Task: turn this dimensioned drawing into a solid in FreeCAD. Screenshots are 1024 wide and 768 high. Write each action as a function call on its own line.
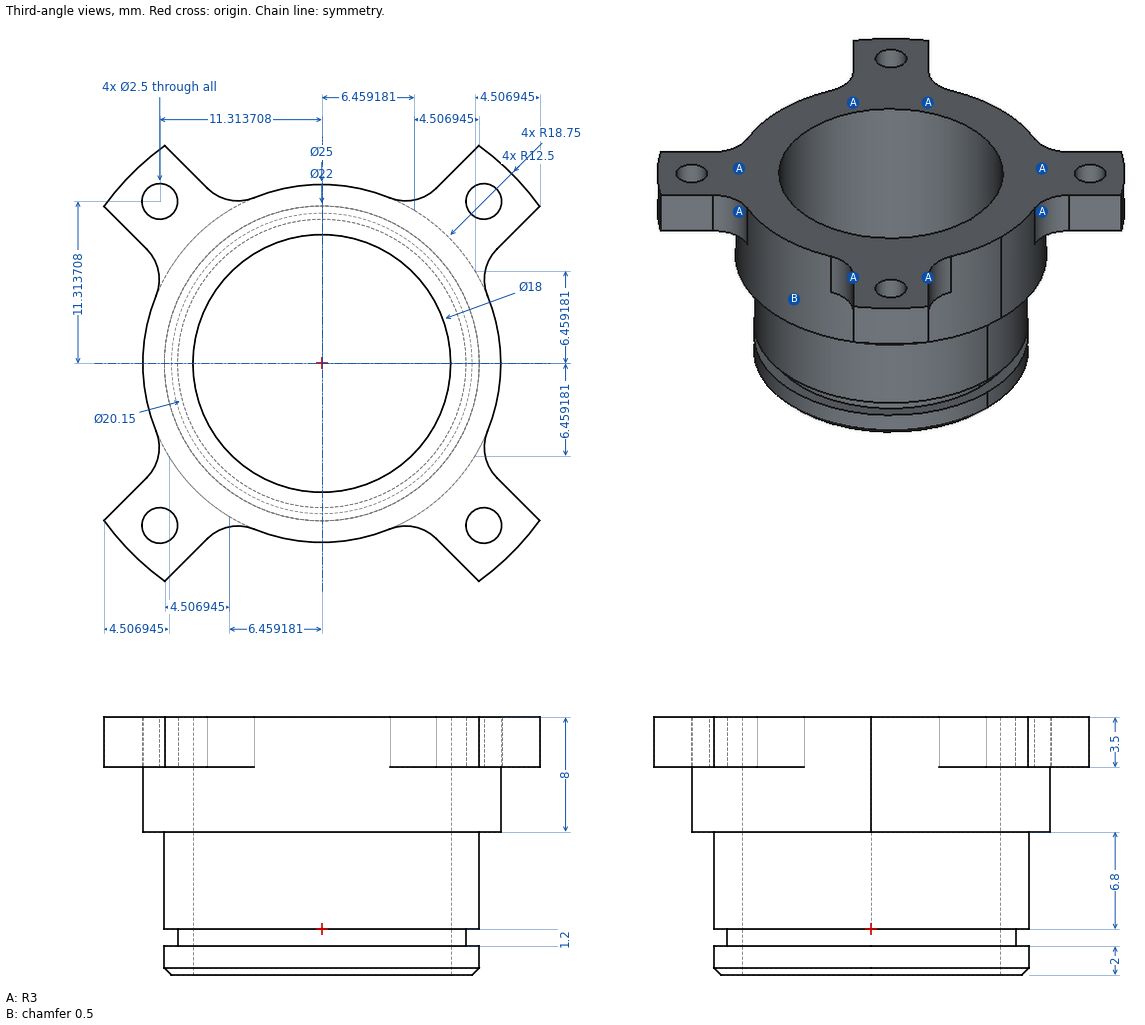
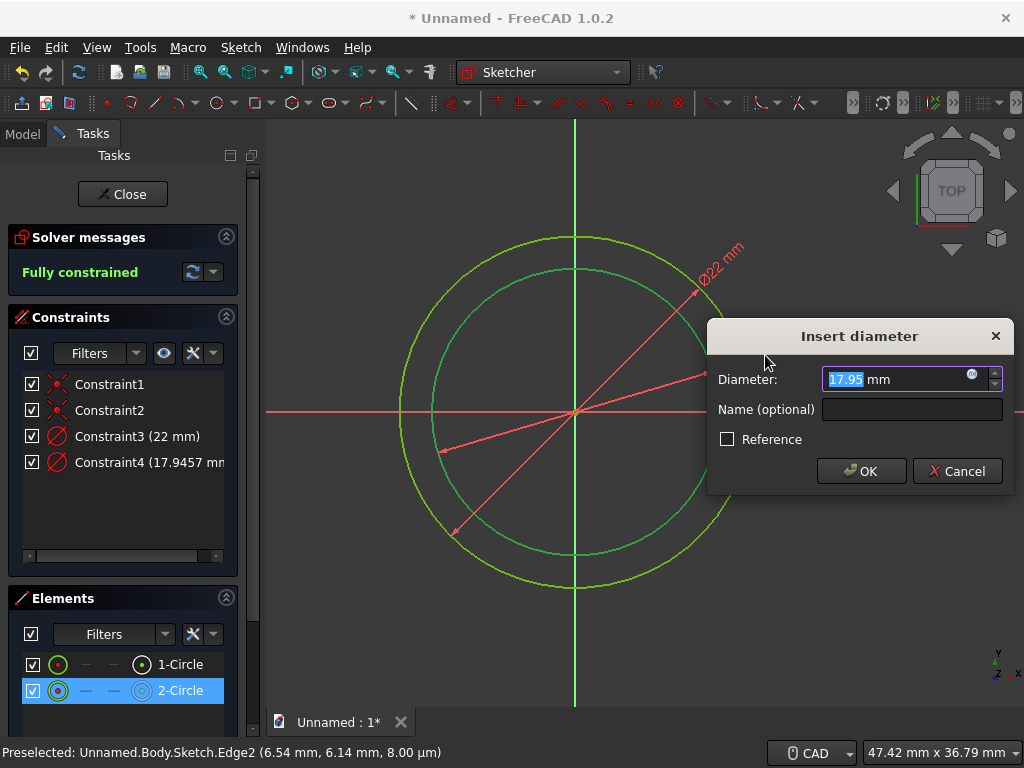
text(18)
key(Return)
key(Escape)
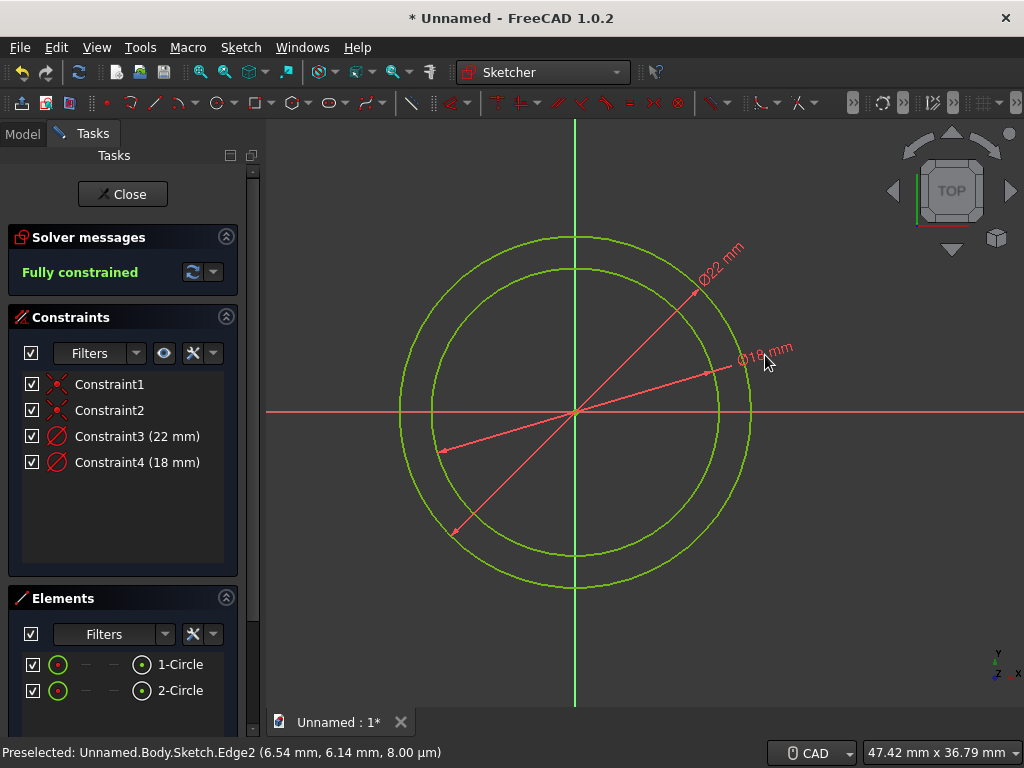
click(123, 194)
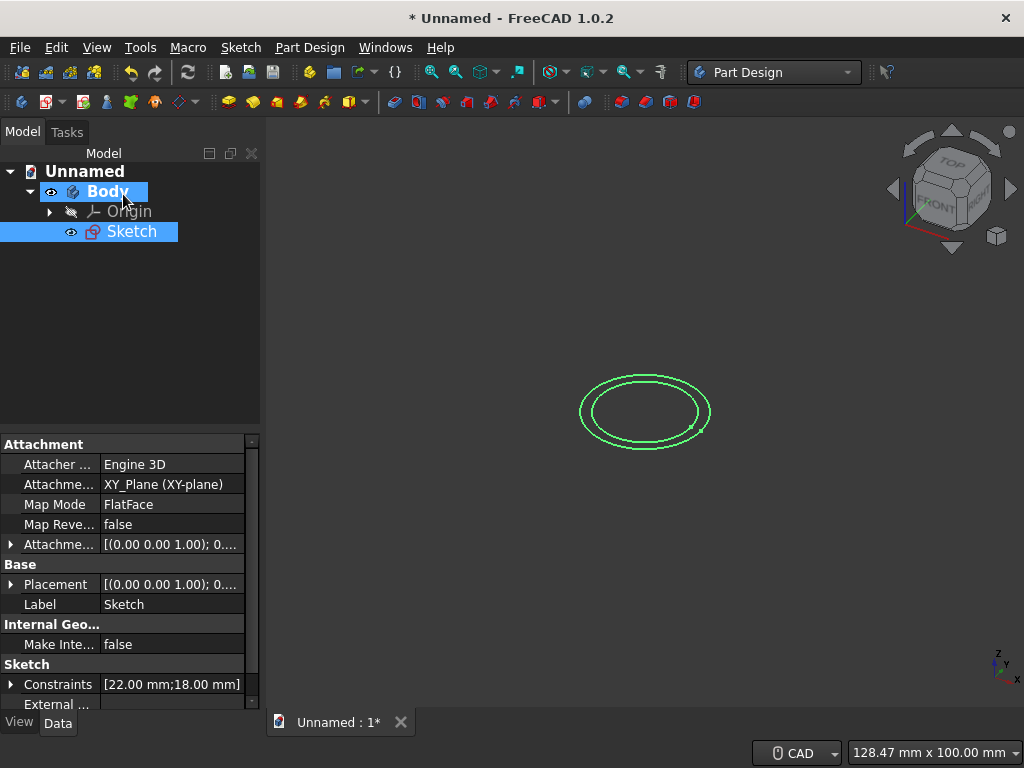
click(230, 102)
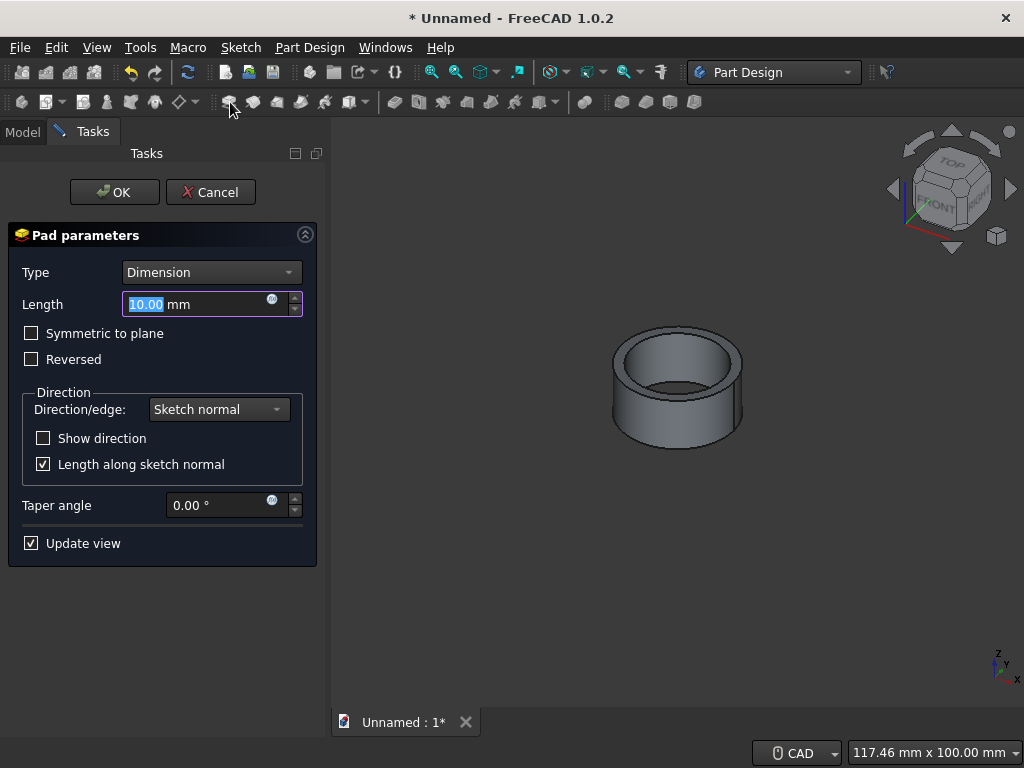
text(6.8)
key(Tab)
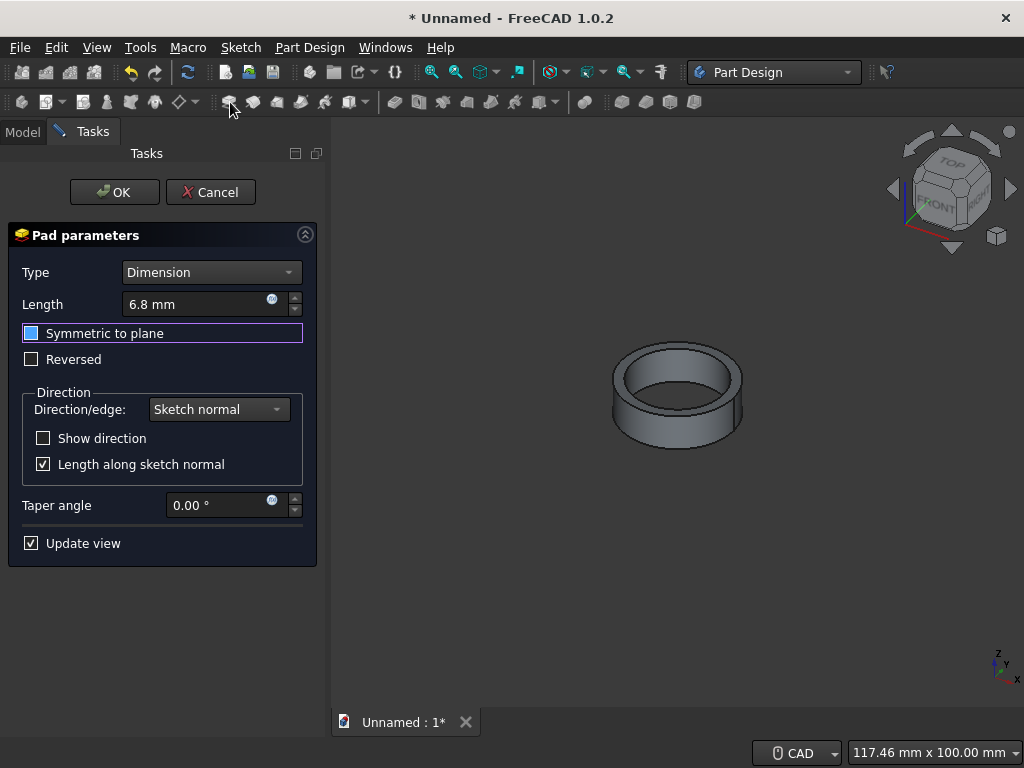
click(115, 192)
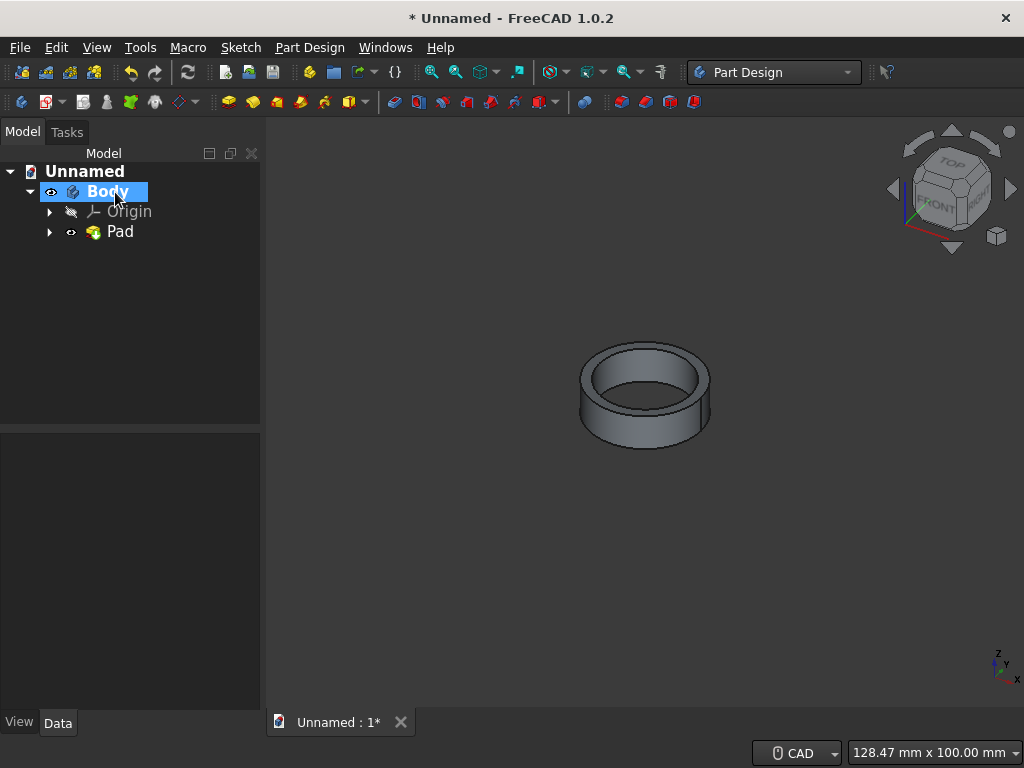
click(432, 72)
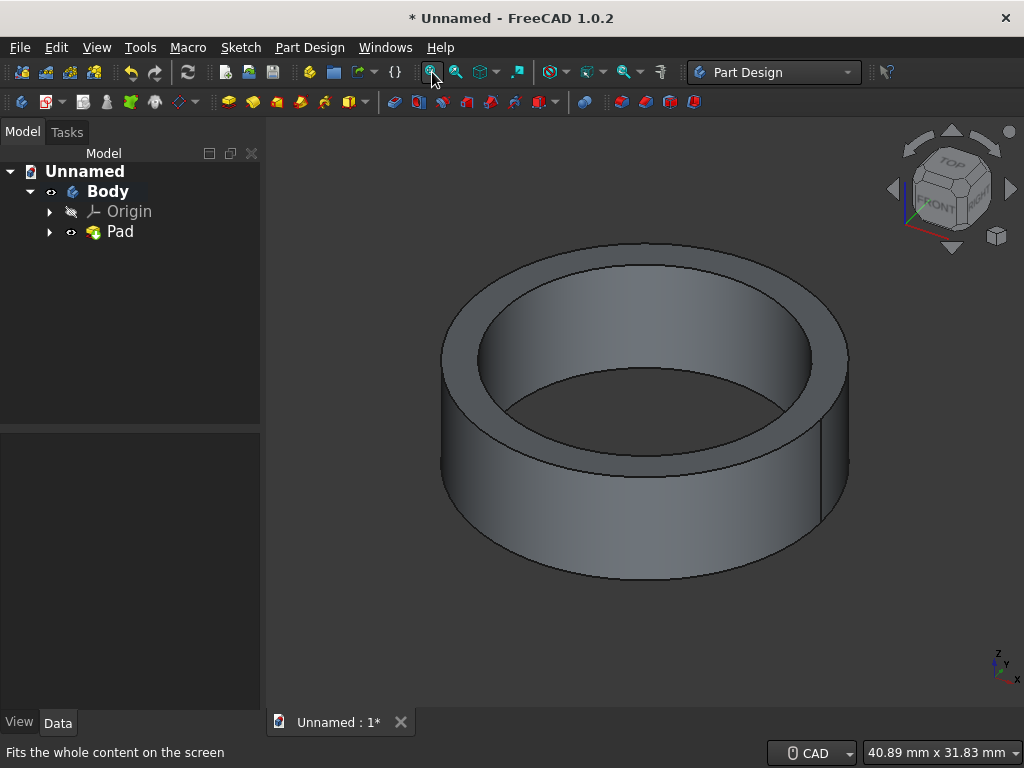
click(507, 429)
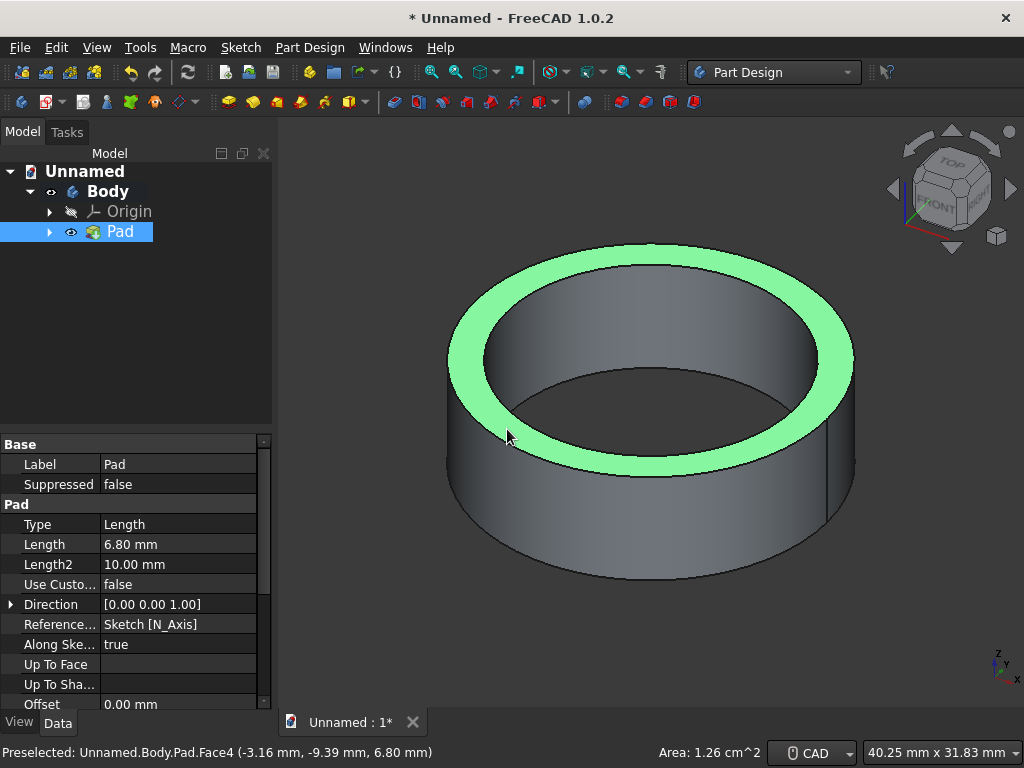
click(46, 102)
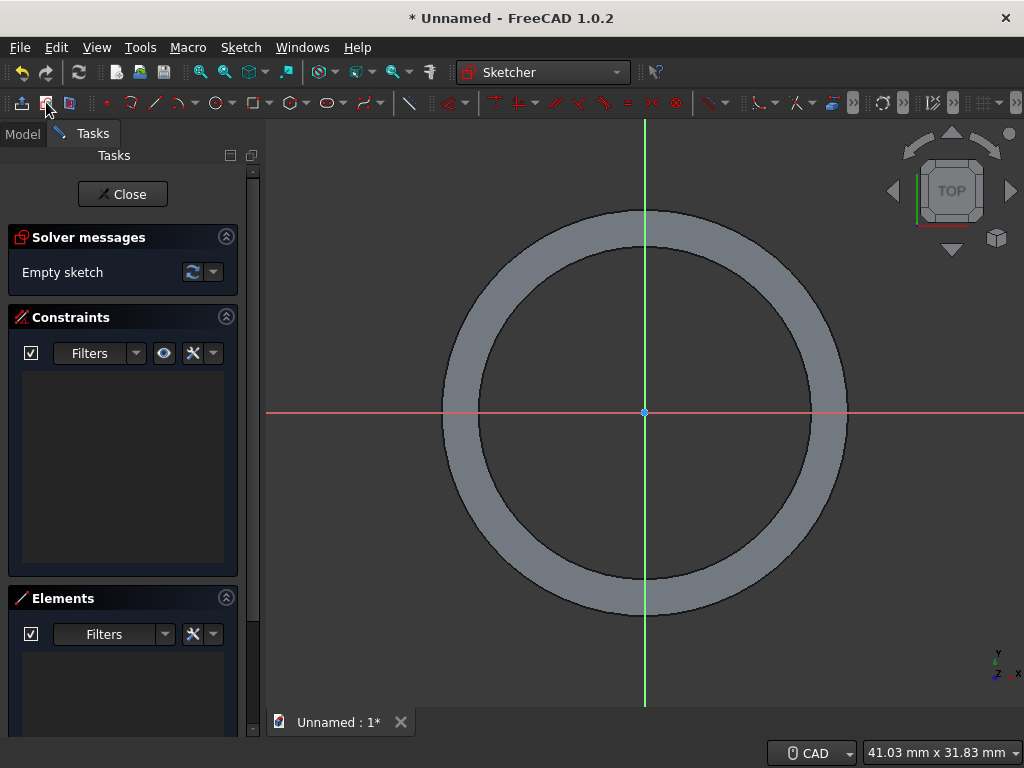
scroll(294, 413, down, 1)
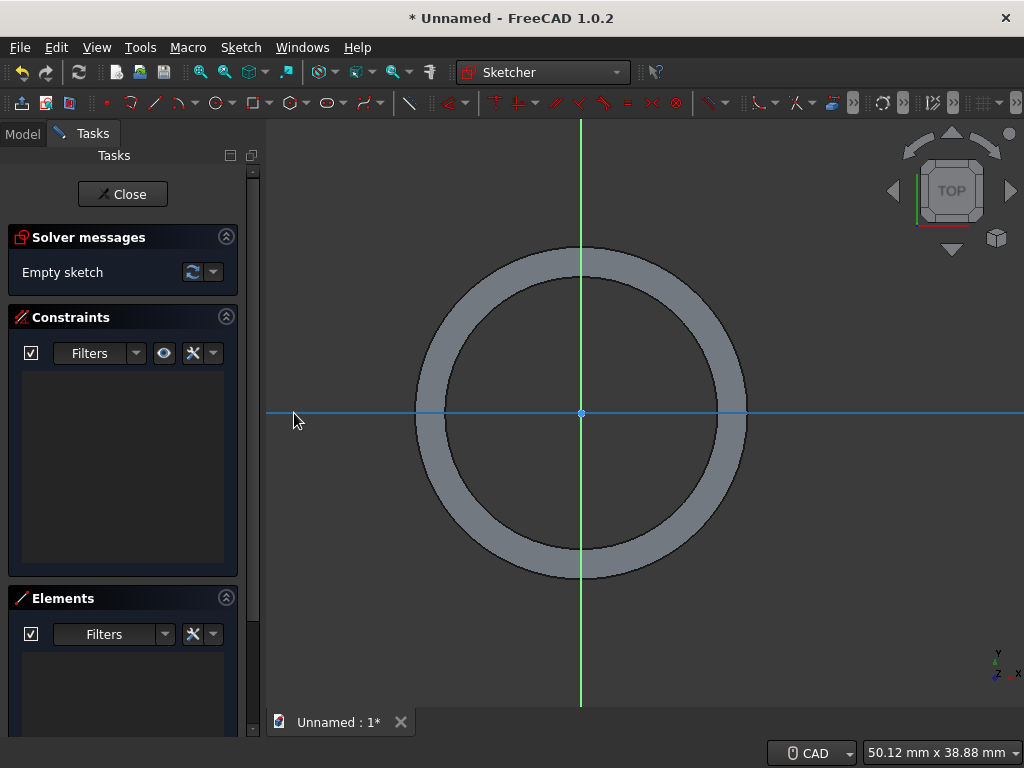
click(216, 104)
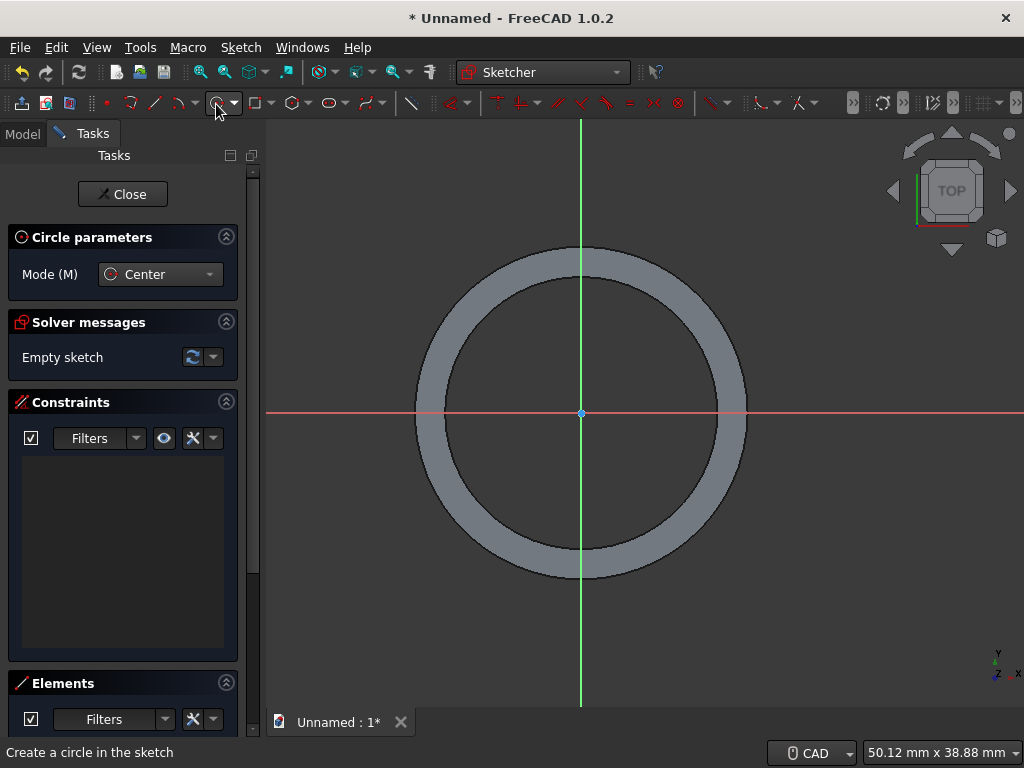
click(581, 413)
click(715, 279)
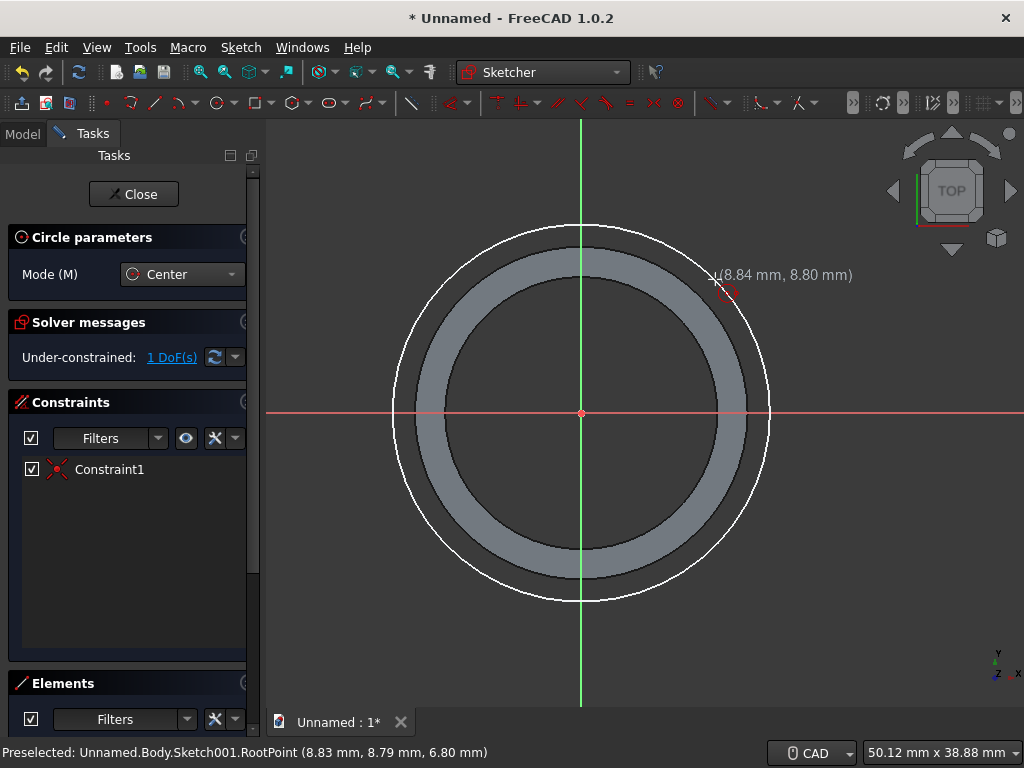
click(581, 413)
click(678, 317)
key(Escape)